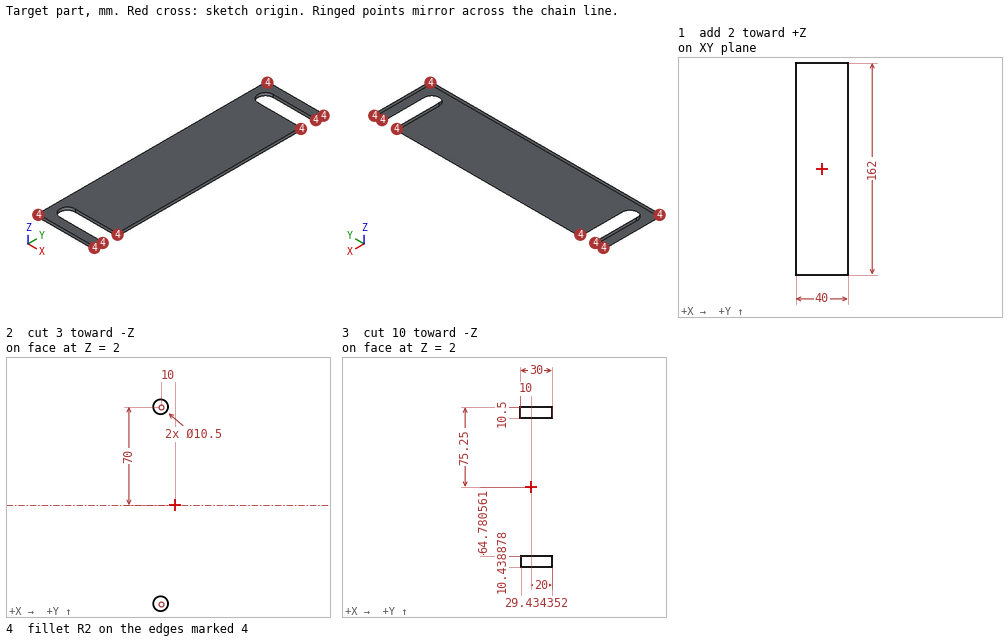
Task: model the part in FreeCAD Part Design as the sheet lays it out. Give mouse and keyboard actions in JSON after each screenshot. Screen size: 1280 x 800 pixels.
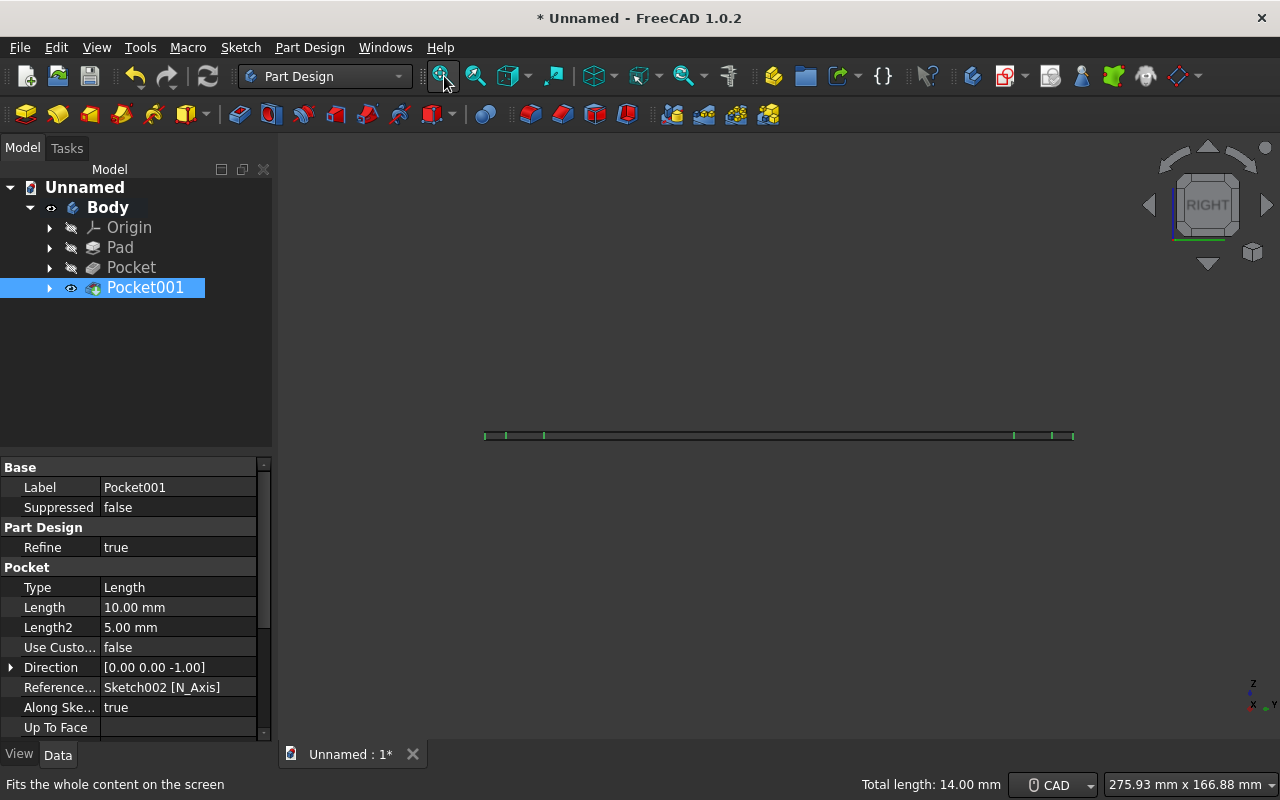
{"action": "scroll", "coordinate": [1073, 435], "scroll_direction": "up", "scroll_amount": 9}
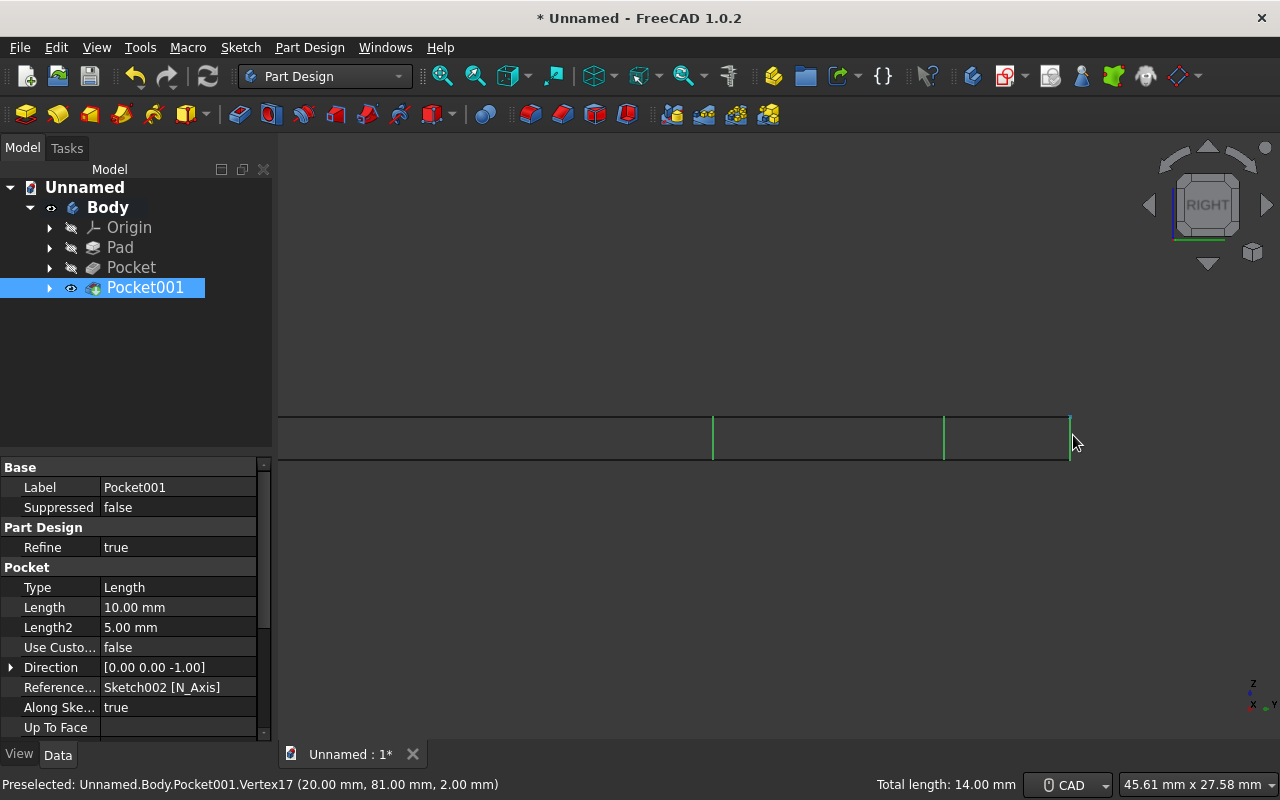
{"action": "left_click", "coordinate": [444, 76]}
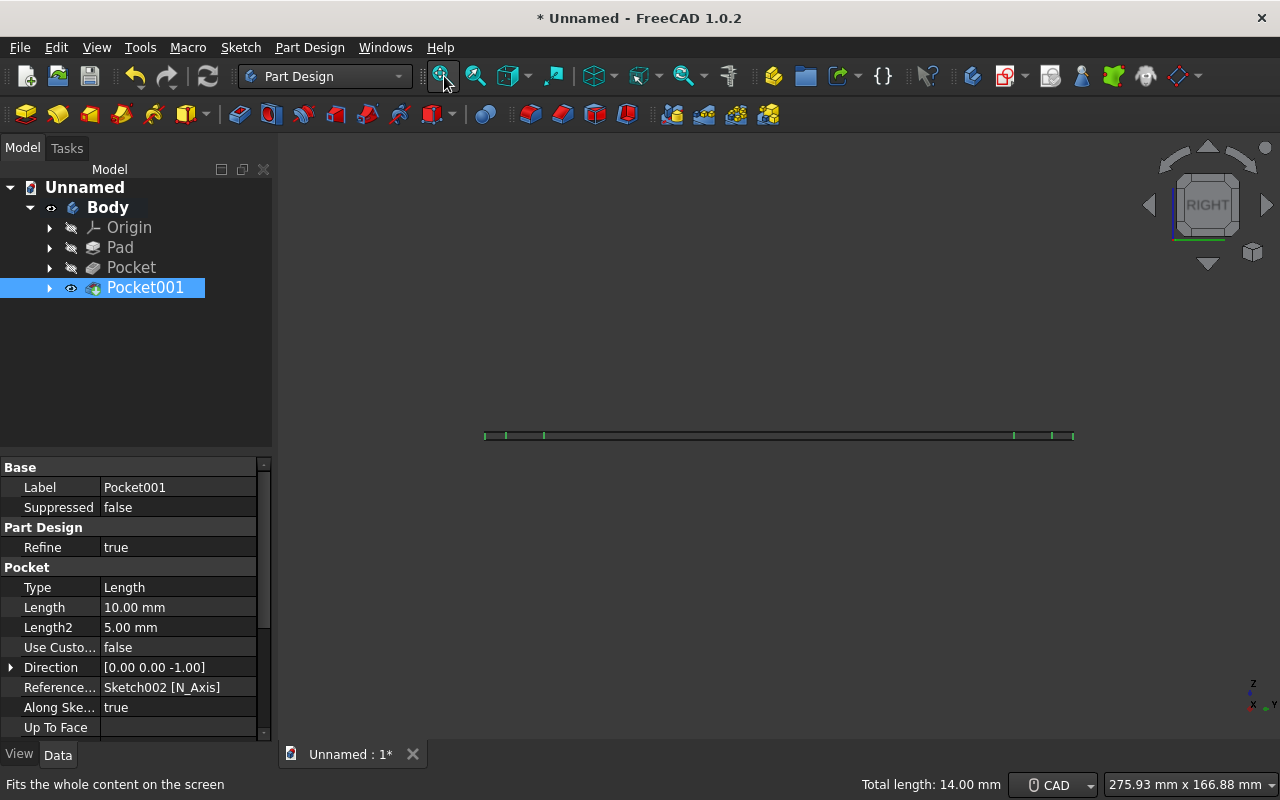
{"action": "key", "text": "5"}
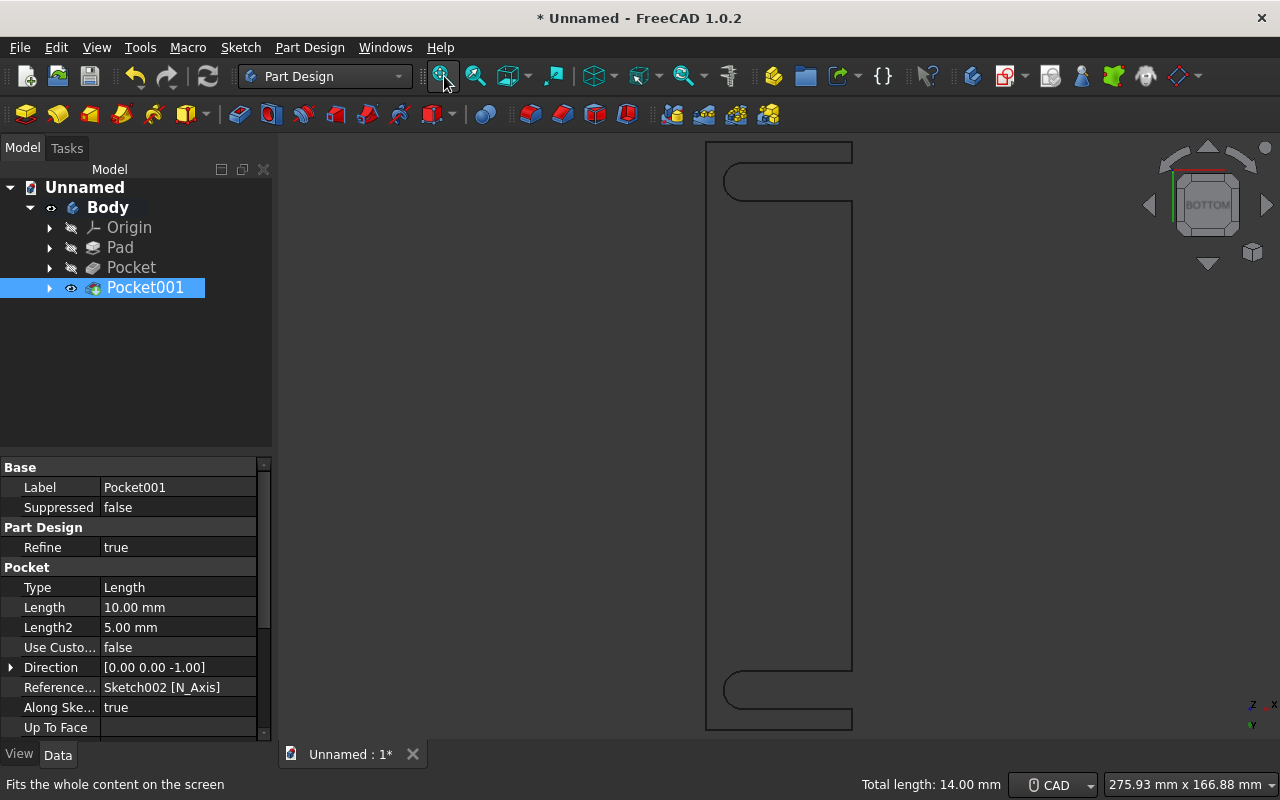
{"action": "key", "text": "4"}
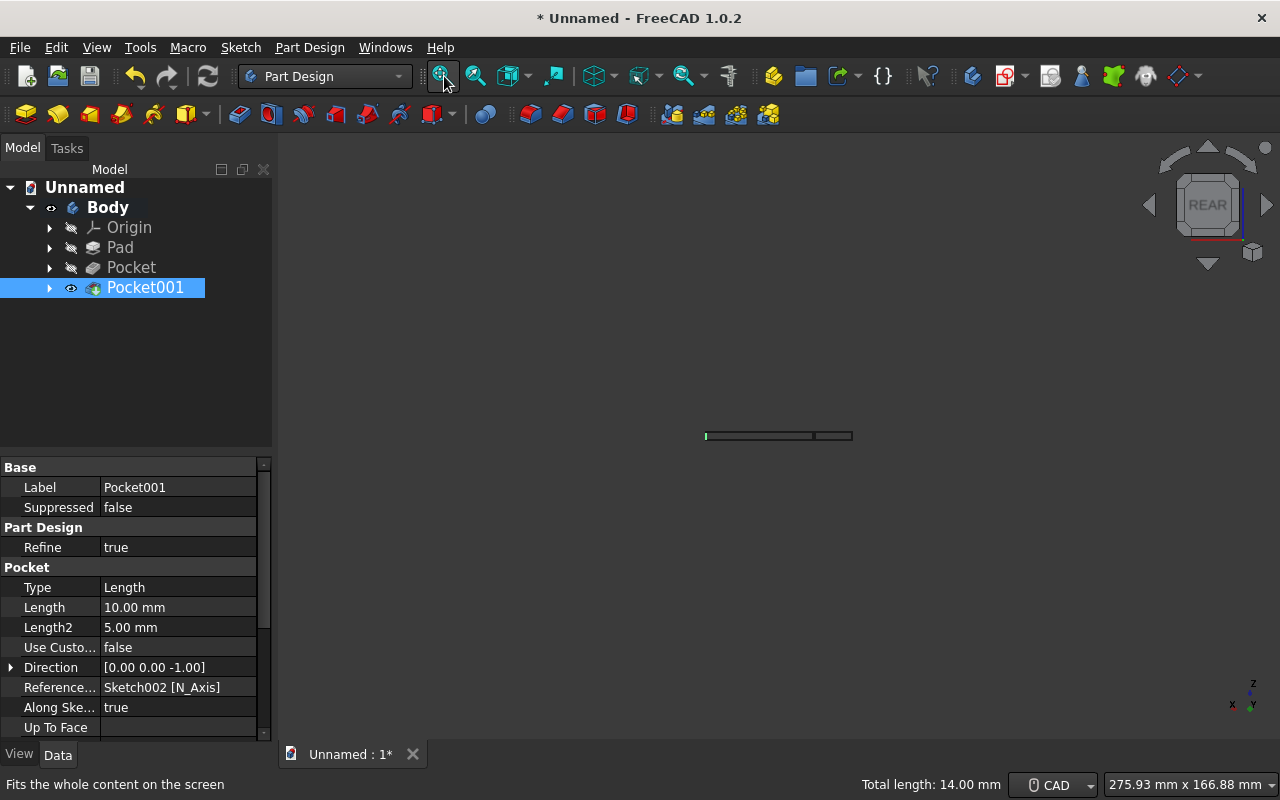
{"action": "left_click", "coordinate": [444, 76]}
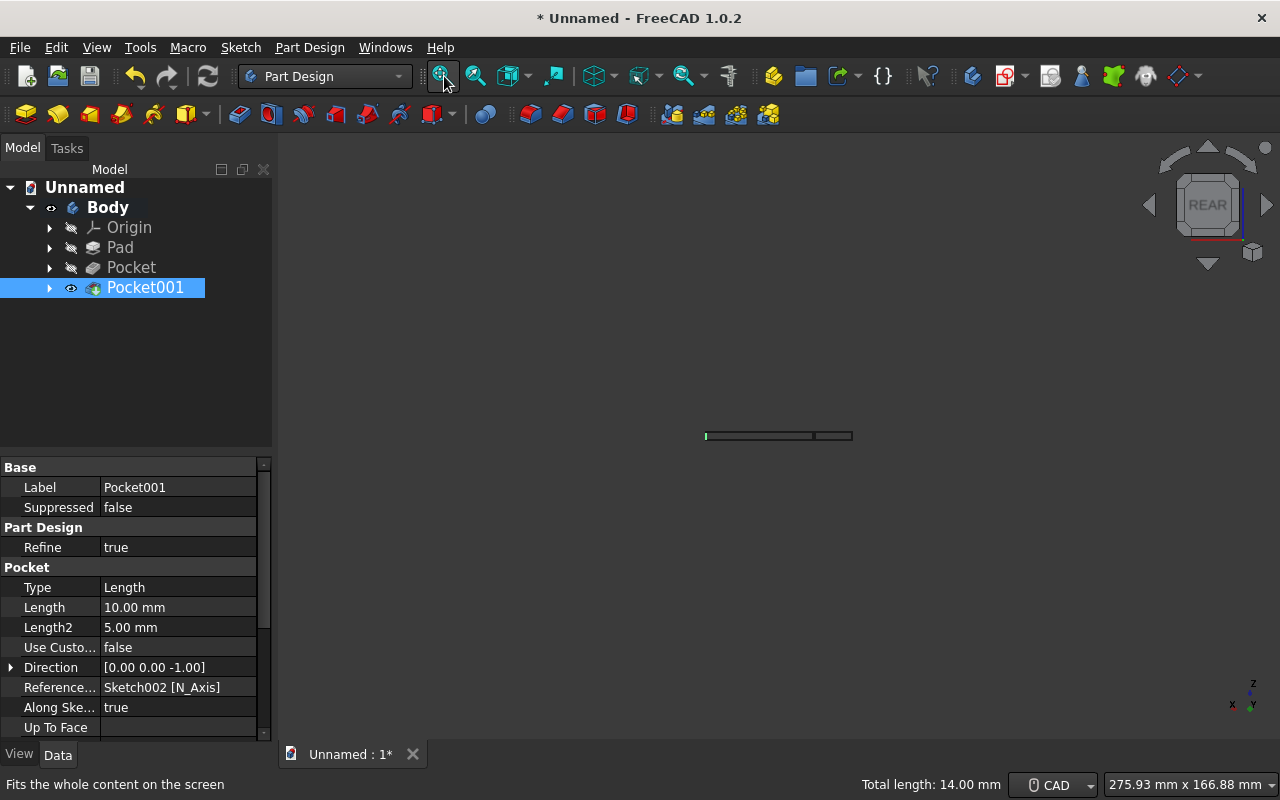
{"action": "scroll", "coordinate": [852, 435], "scroll_direction": "up", "scroll_amount": 9}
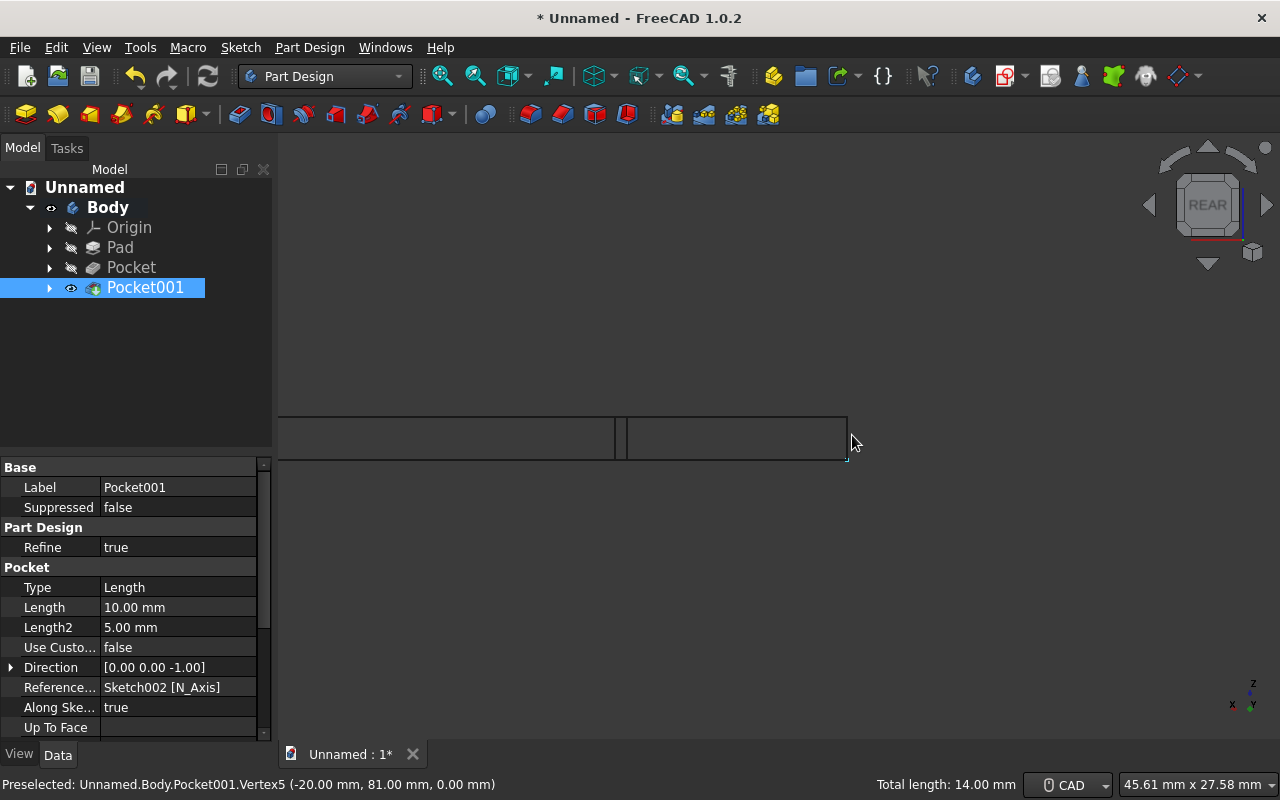
{"action": "left_click", "coordinate": [847, 438], "text": "ctrl"}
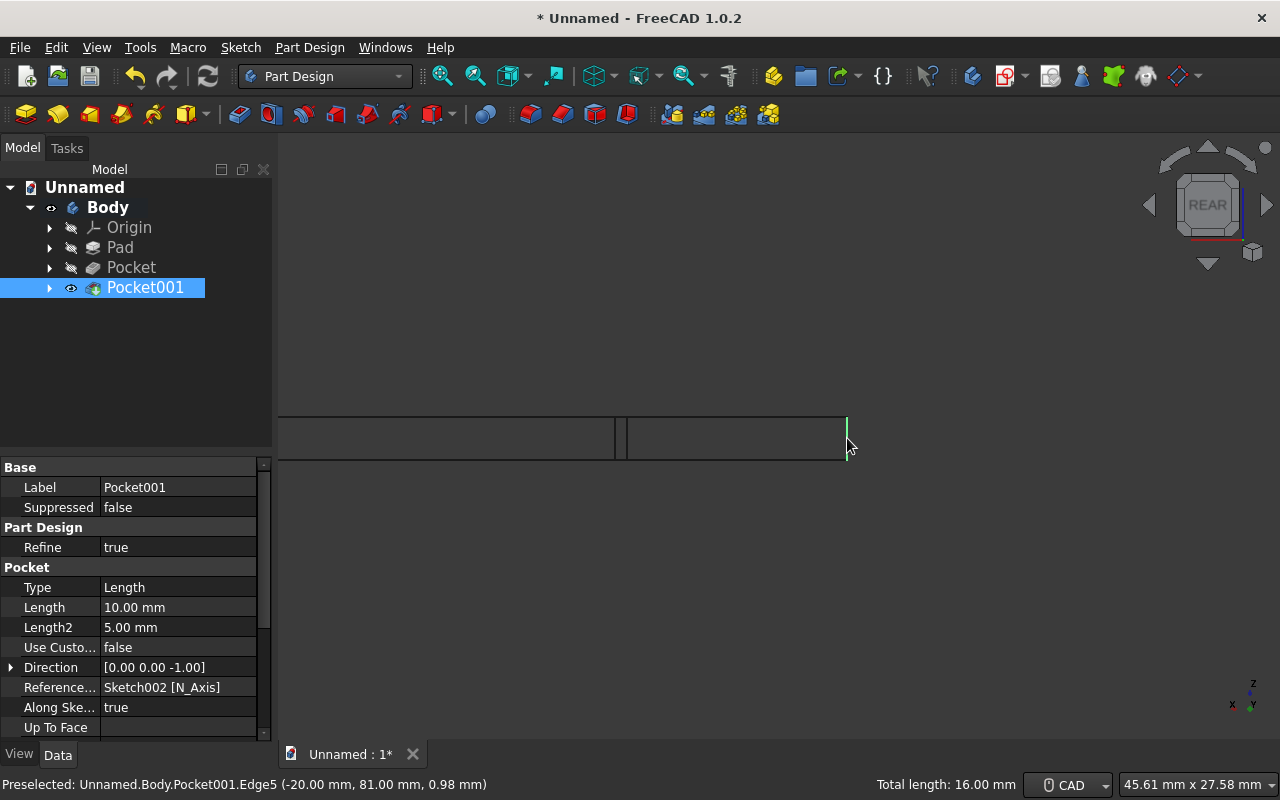
{"action": "key", "text": "v 1"}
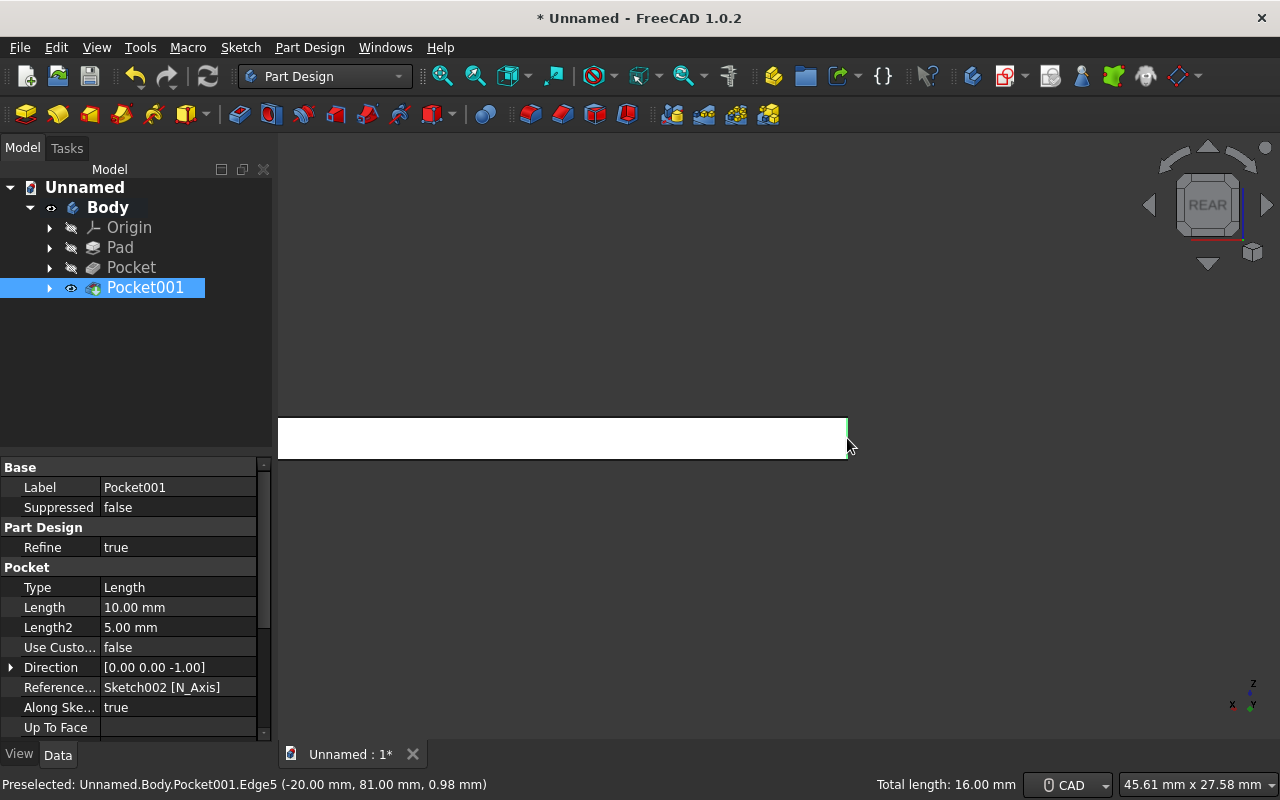
{"action": "left_click", "coordinate": [532, 114]}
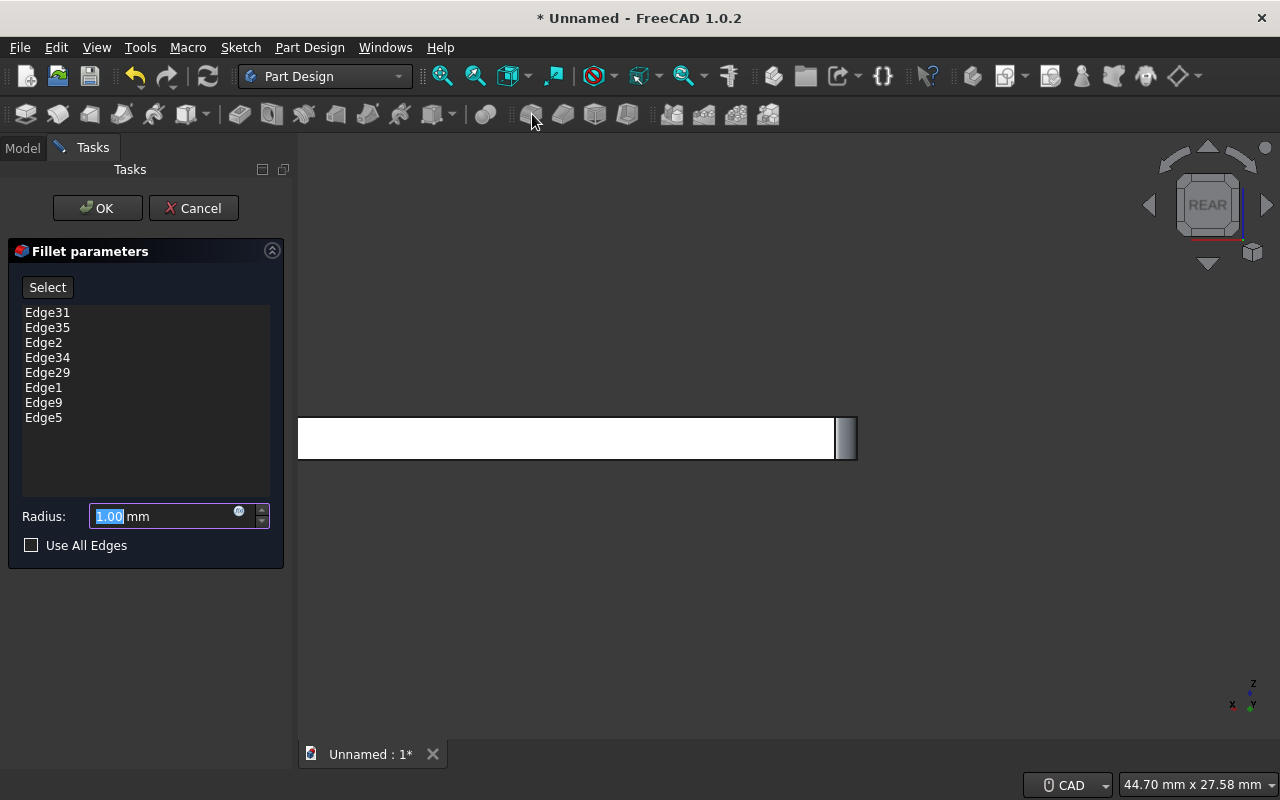
{"action": "type", "text": "2"}
{"action": "key", "text": "Tab"}